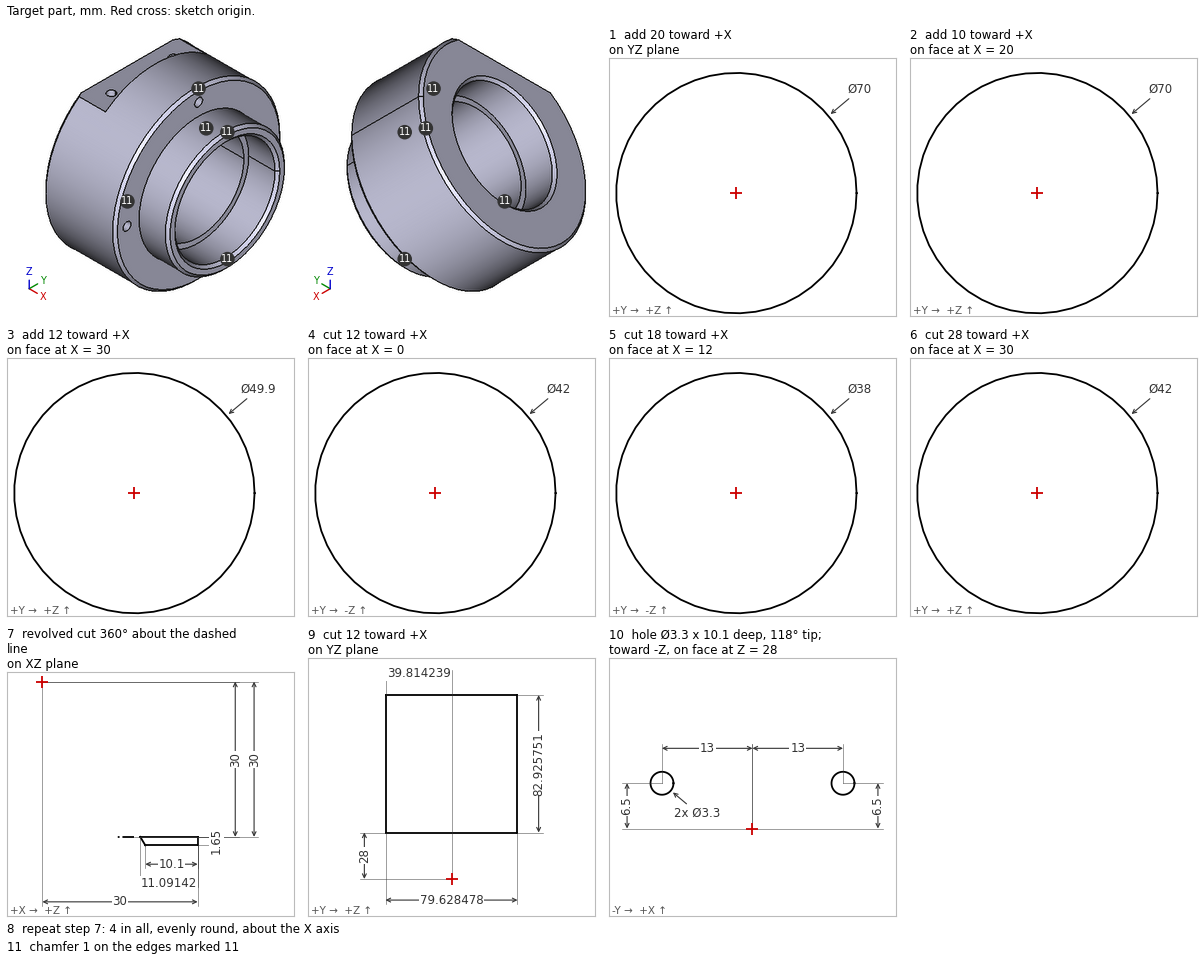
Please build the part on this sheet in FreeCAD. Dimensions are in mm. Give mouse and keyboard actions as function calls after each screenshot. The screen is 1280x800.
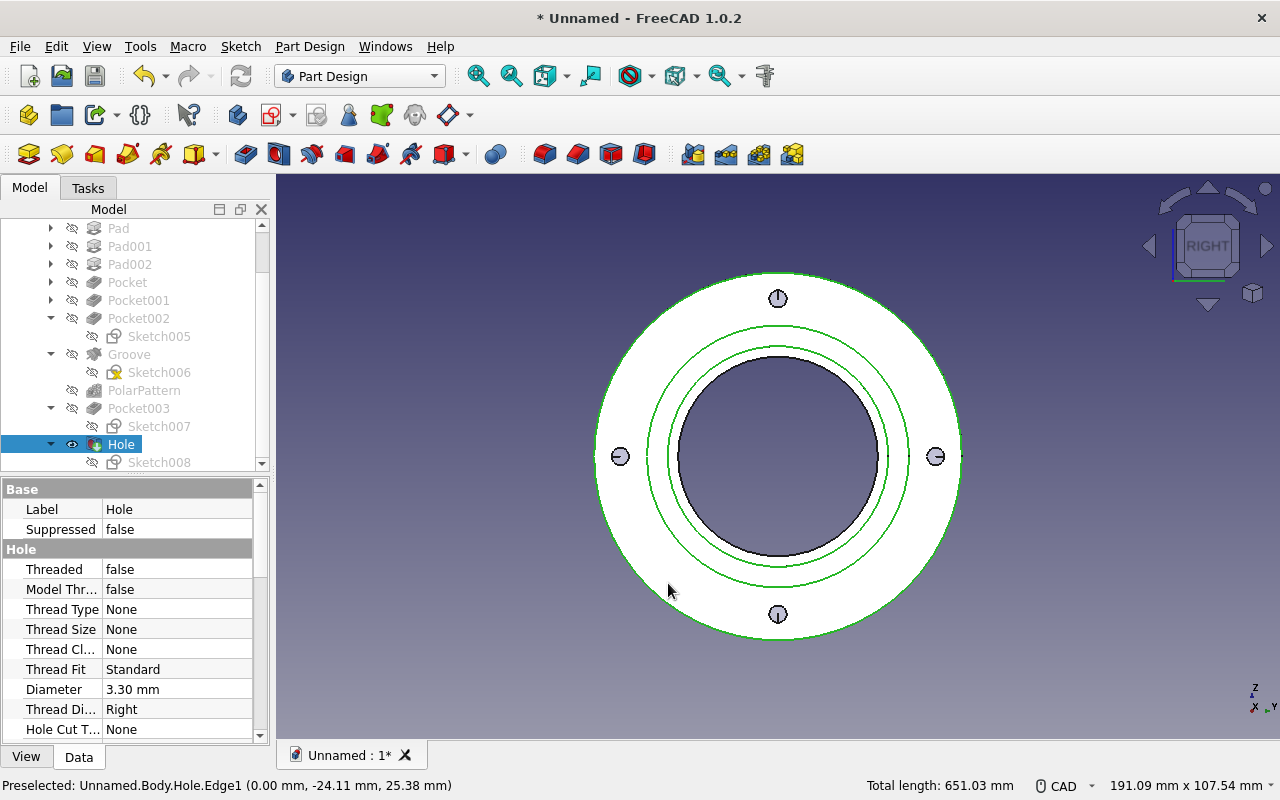
key(5)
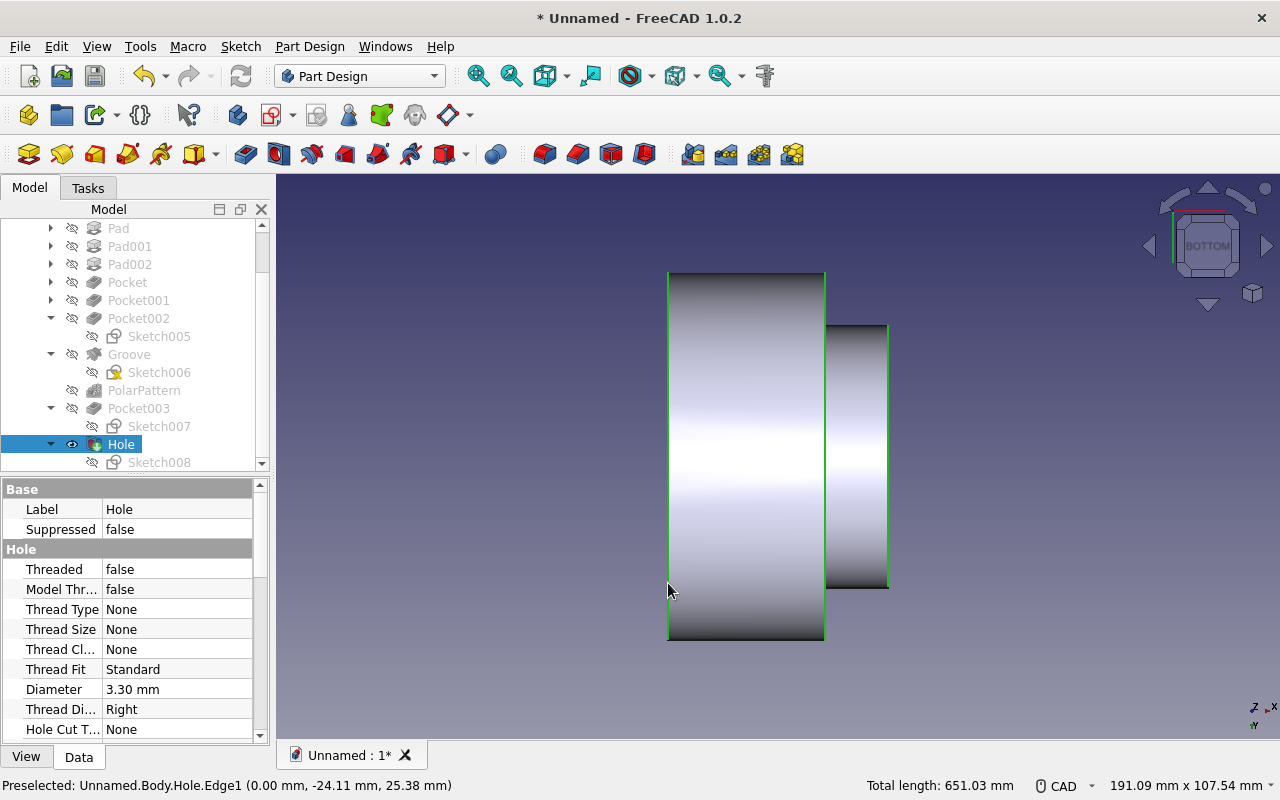
key(4)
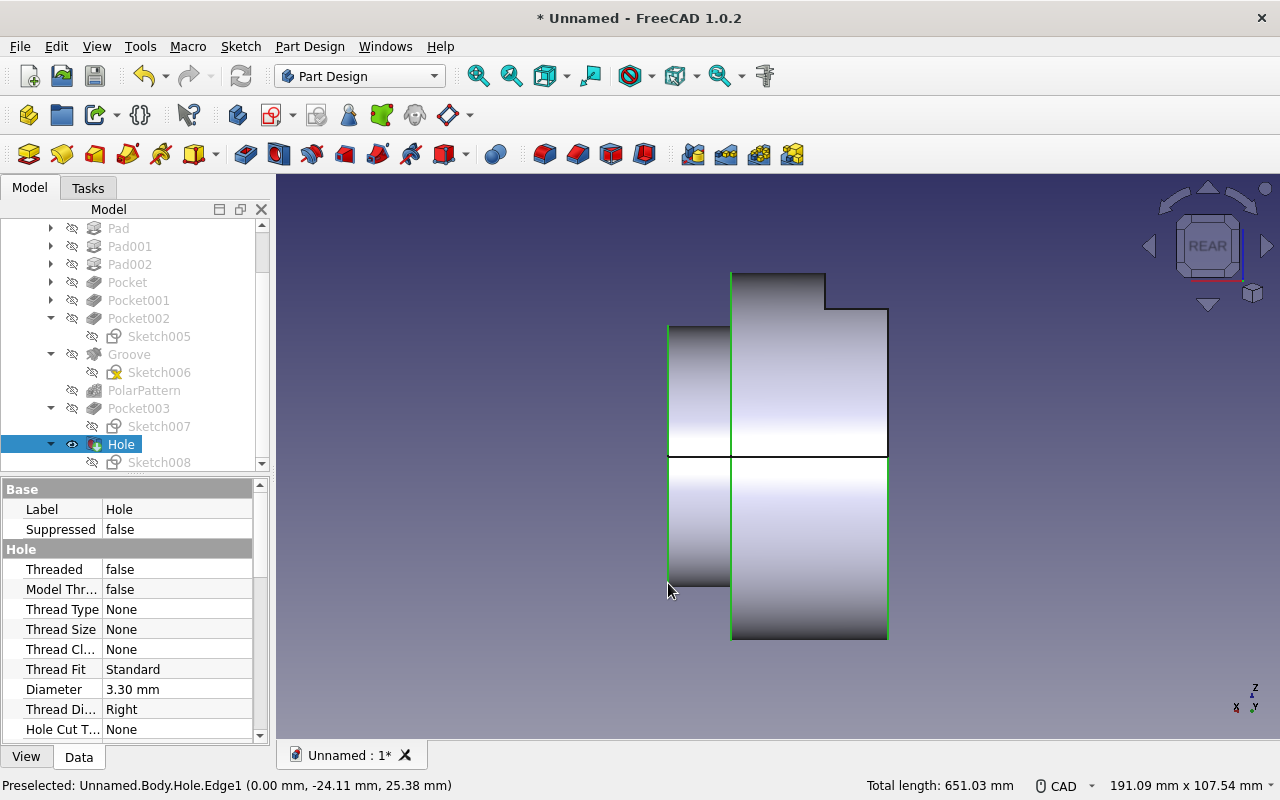
key(6)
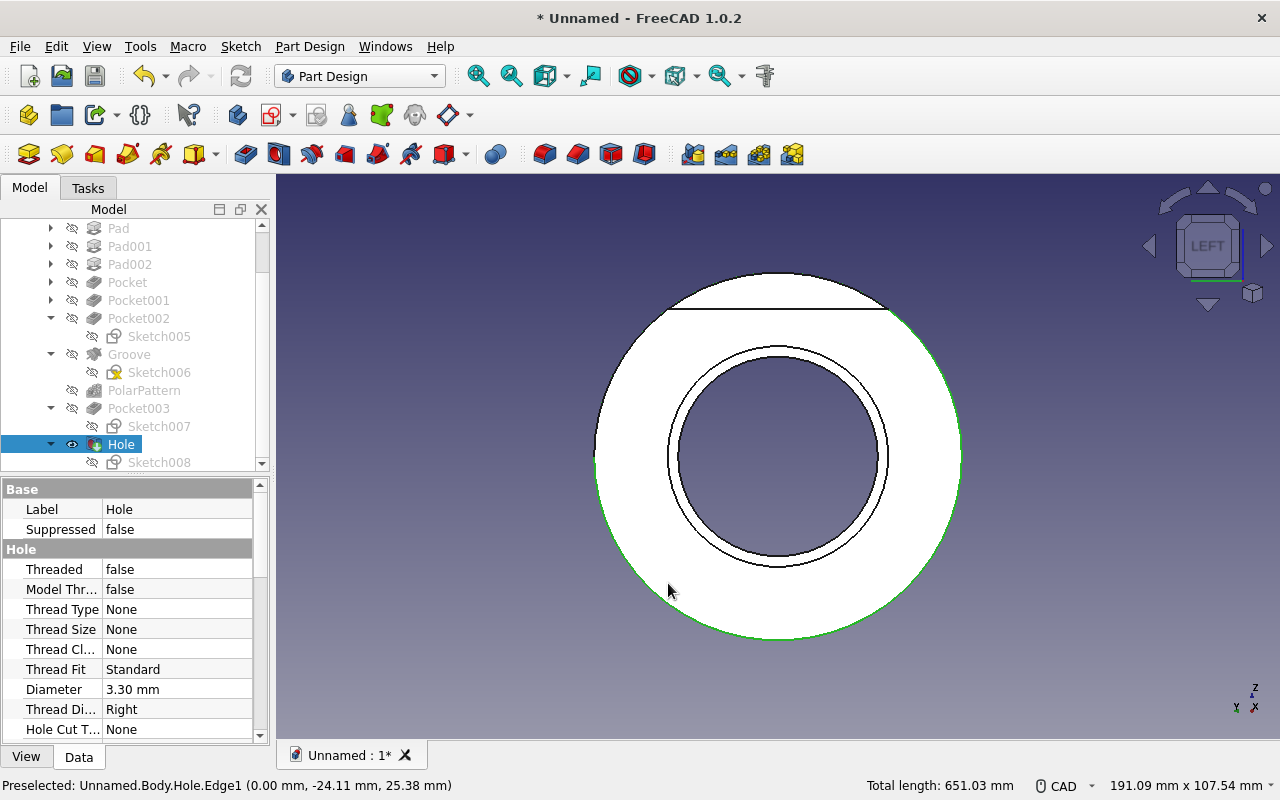
click(867, 520, ctrl)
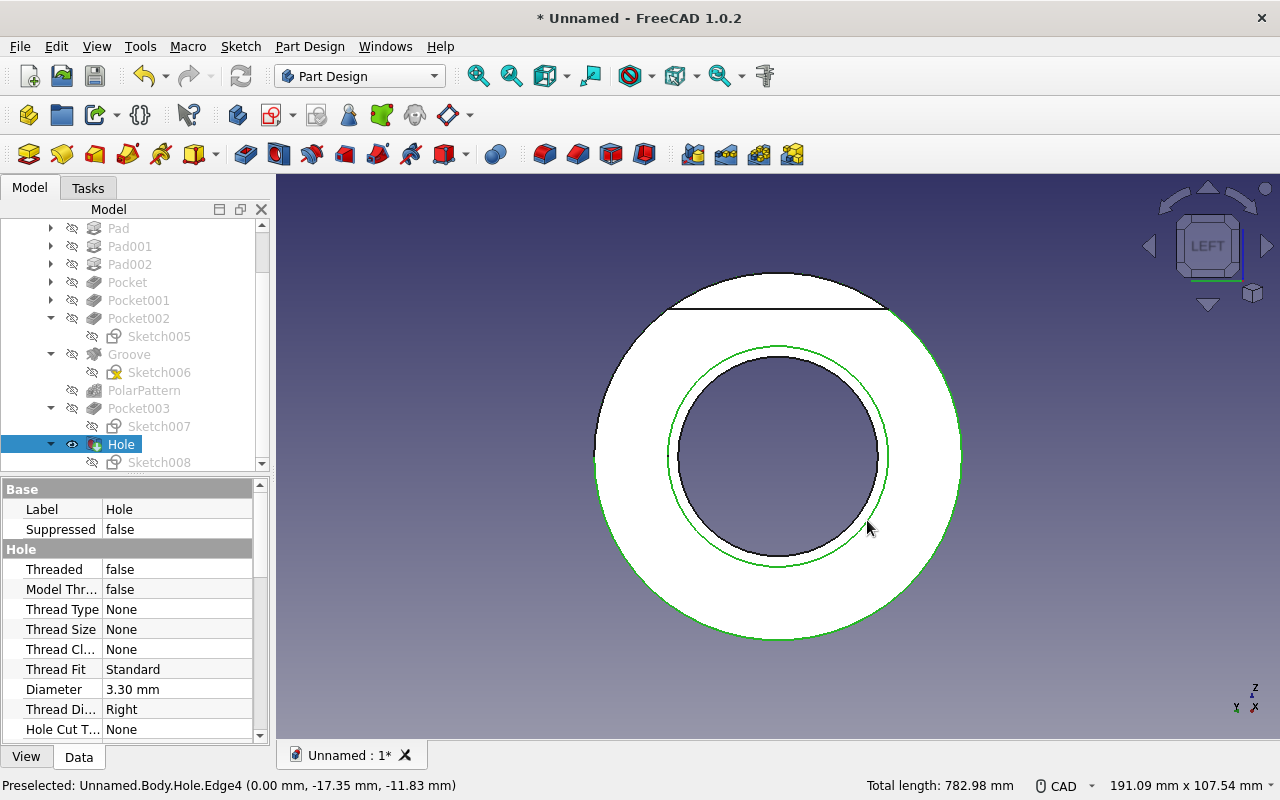
click(578, 154)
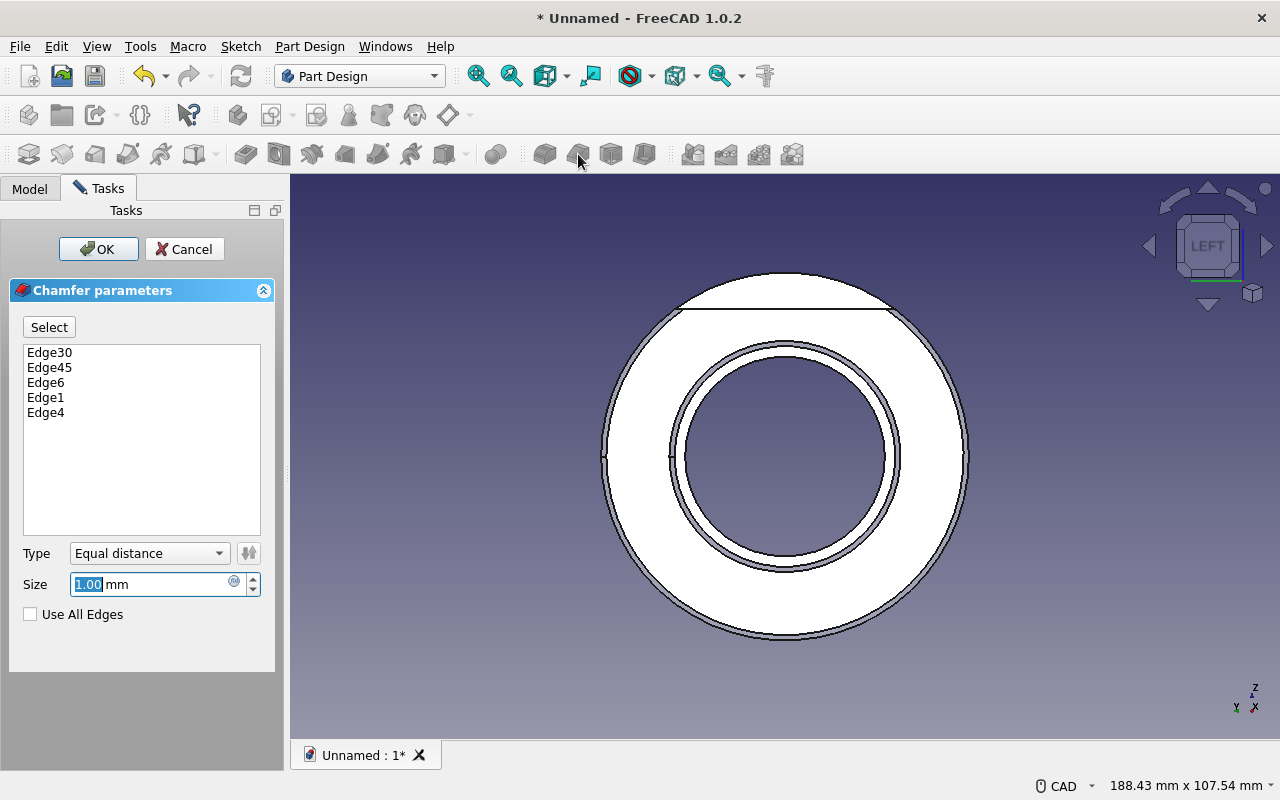
text(1)
key(Tab)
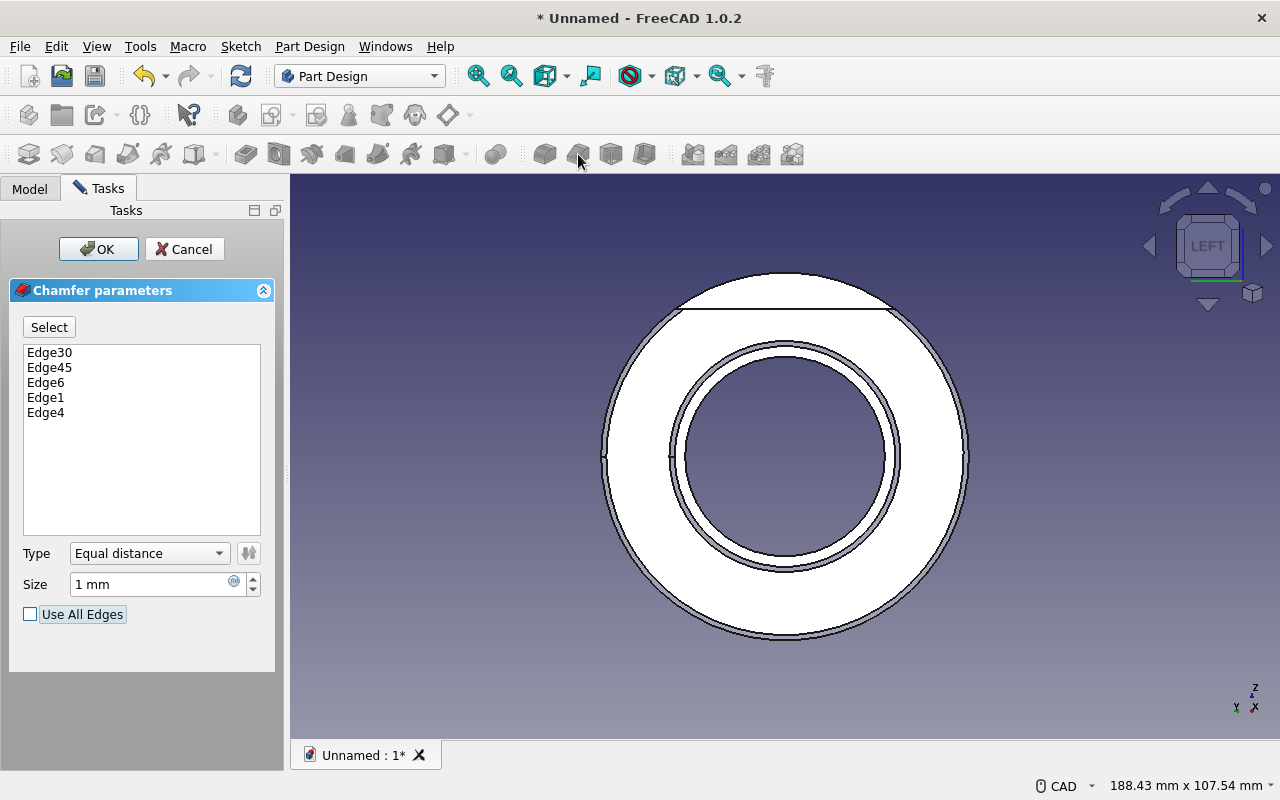
click(99, 249)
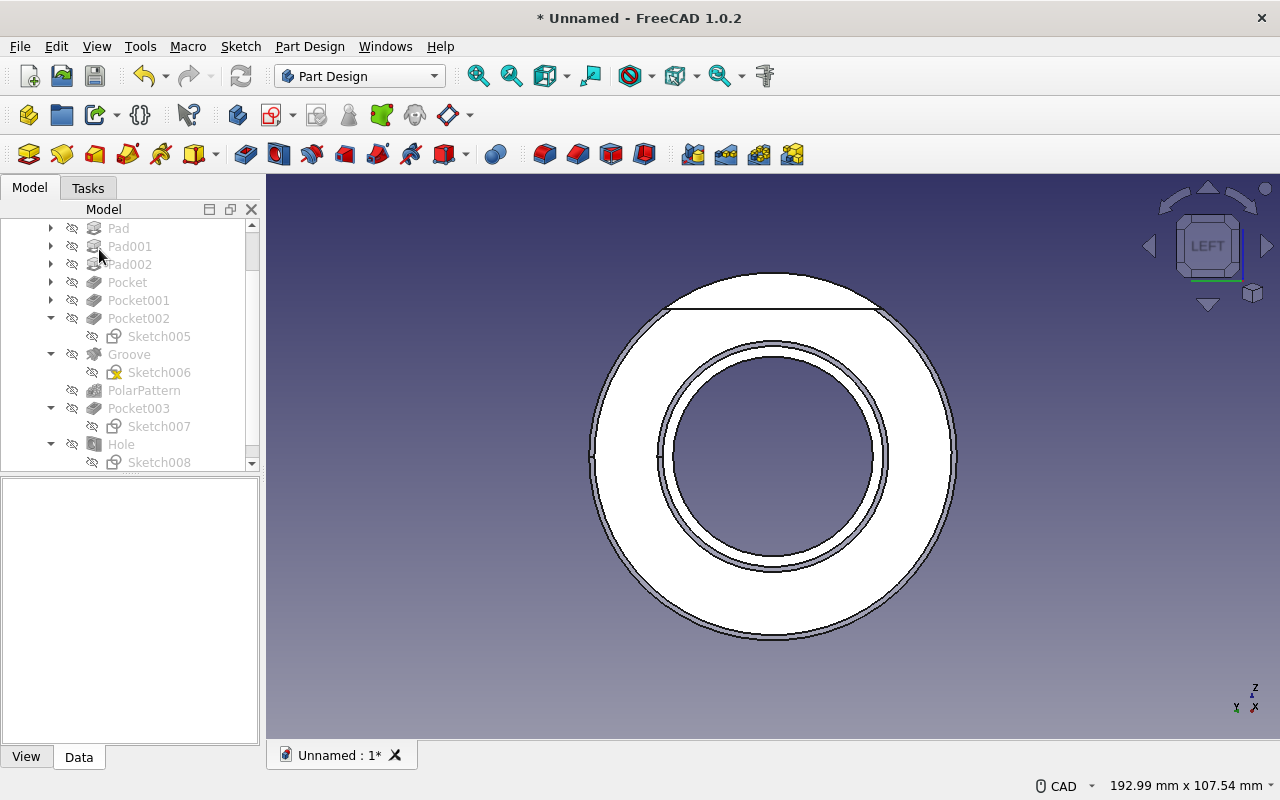
key(0)